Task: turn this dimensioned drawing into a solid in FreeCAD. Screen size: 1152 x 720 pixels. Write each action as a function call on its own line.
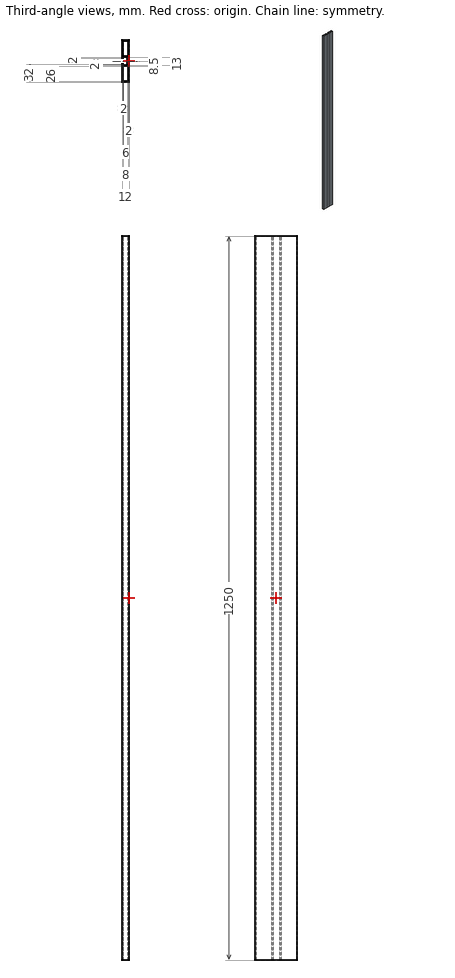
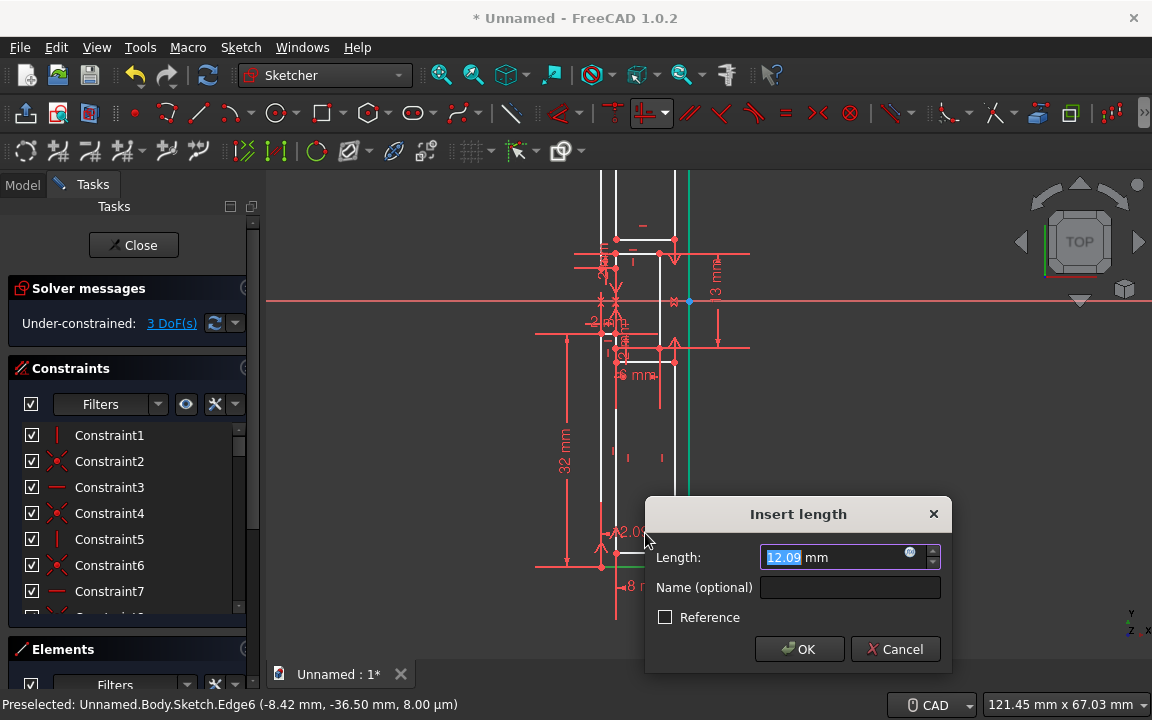
text(12)
key(Return)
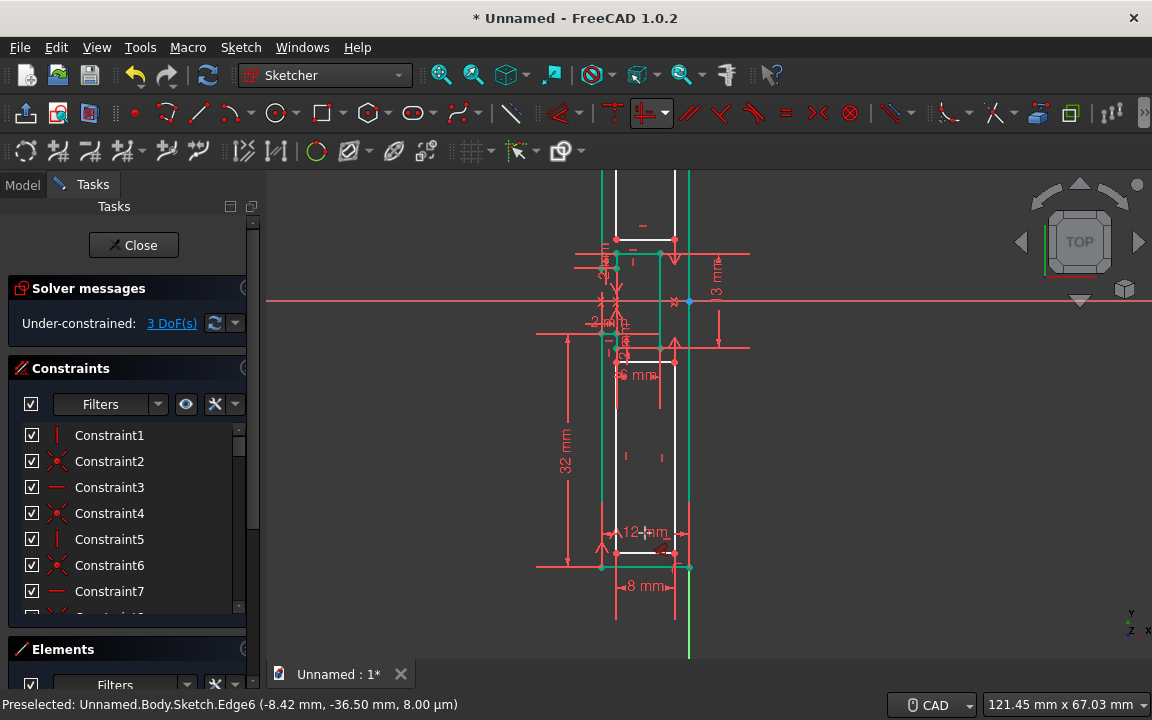
click(616, 420)
click(582, 414)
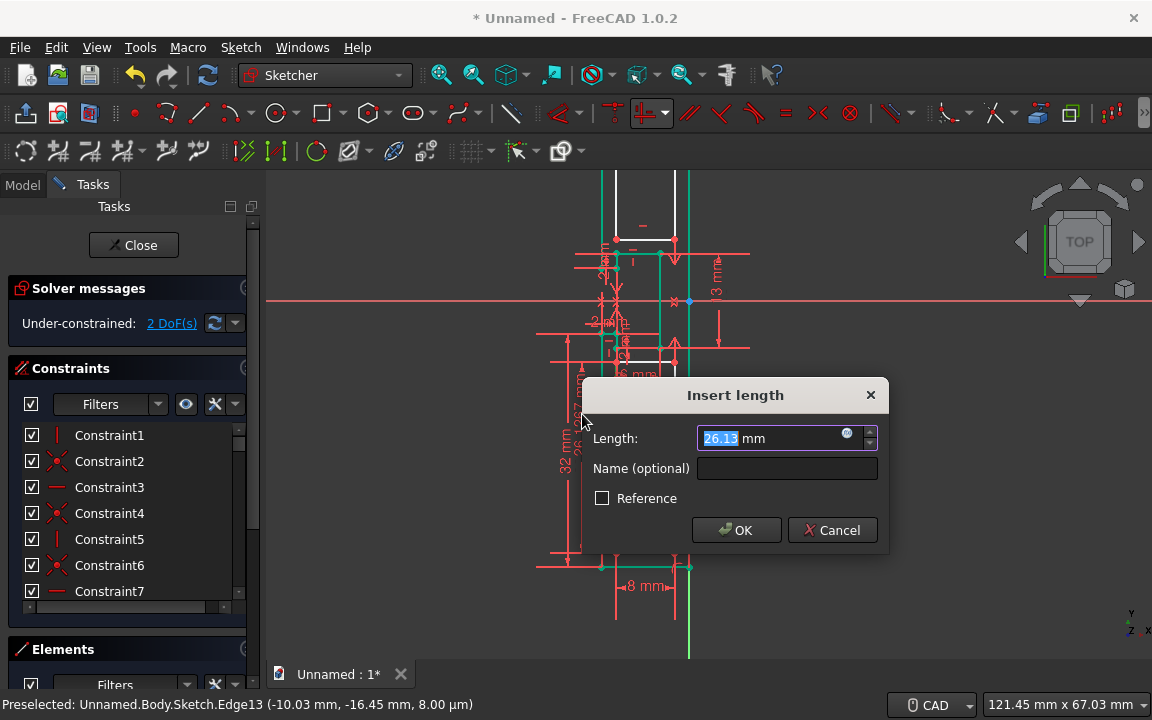
text(26)
key(Return)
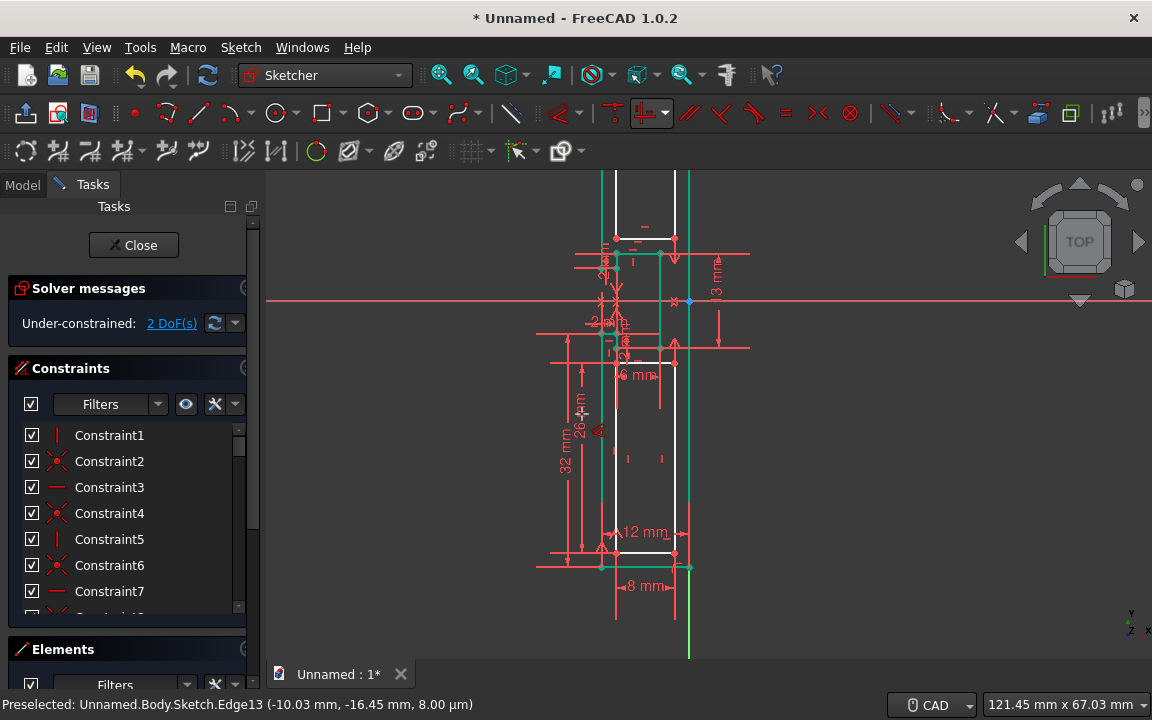
scroll(675, 553, up, 6)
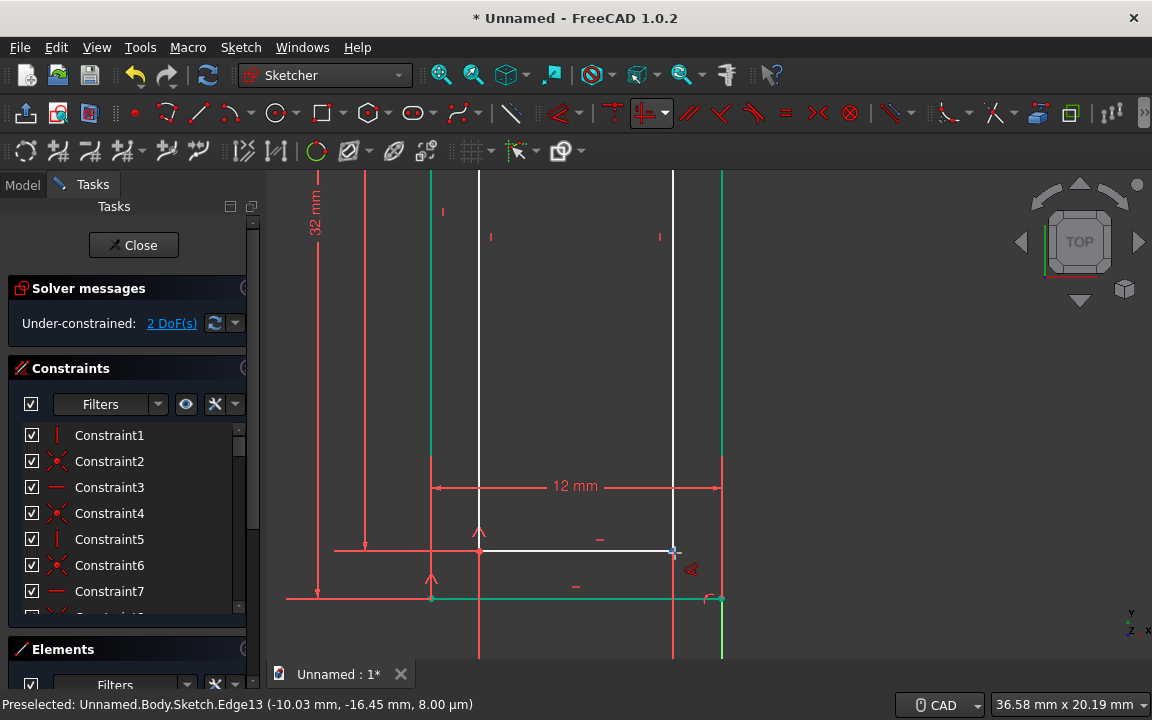
click(673, 551)
click(697, 585)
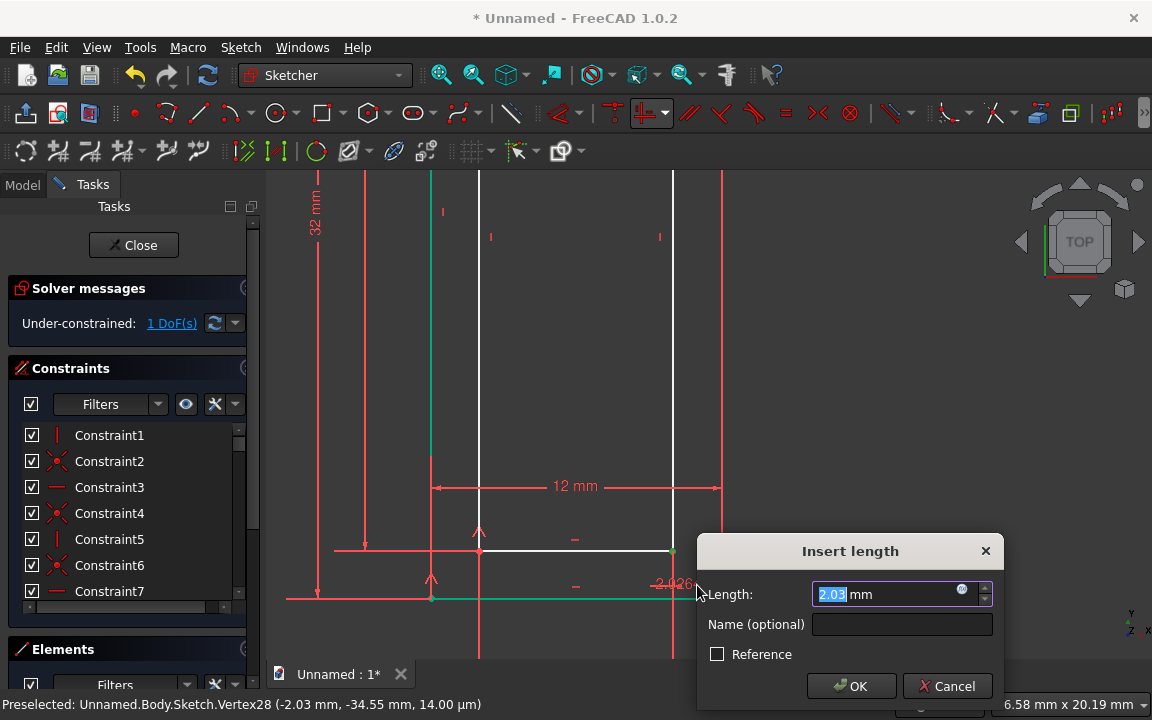
text(2)
key(Return)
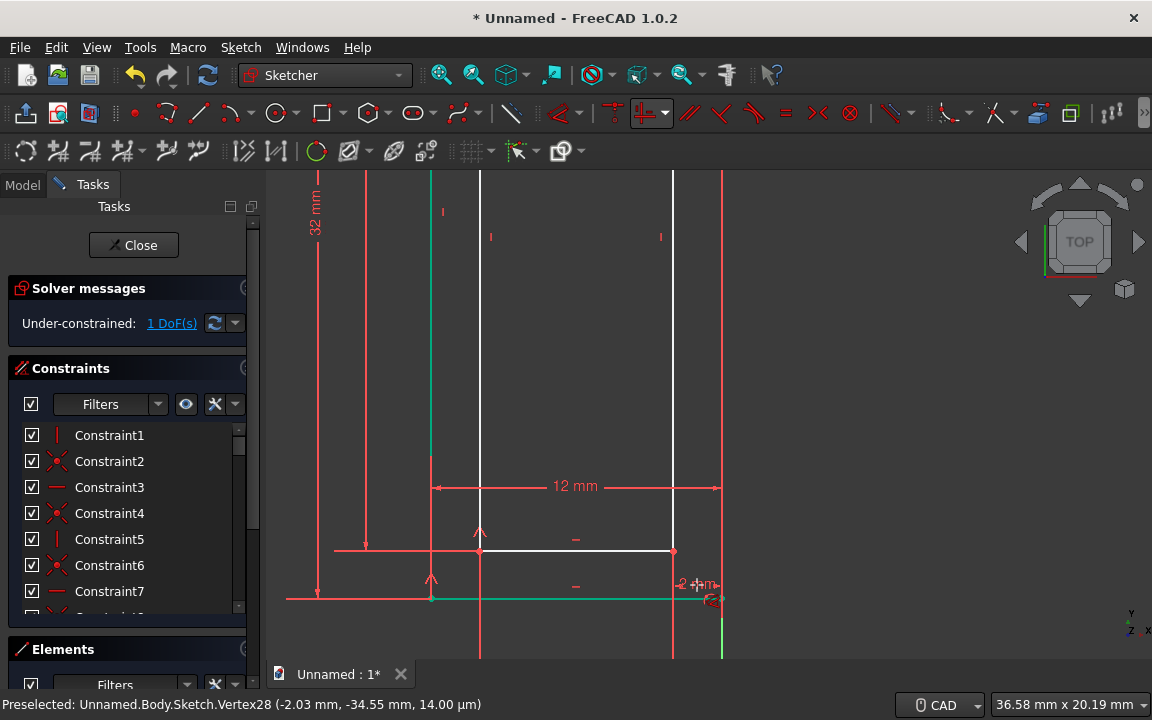
scroll(653, 553, down, 9)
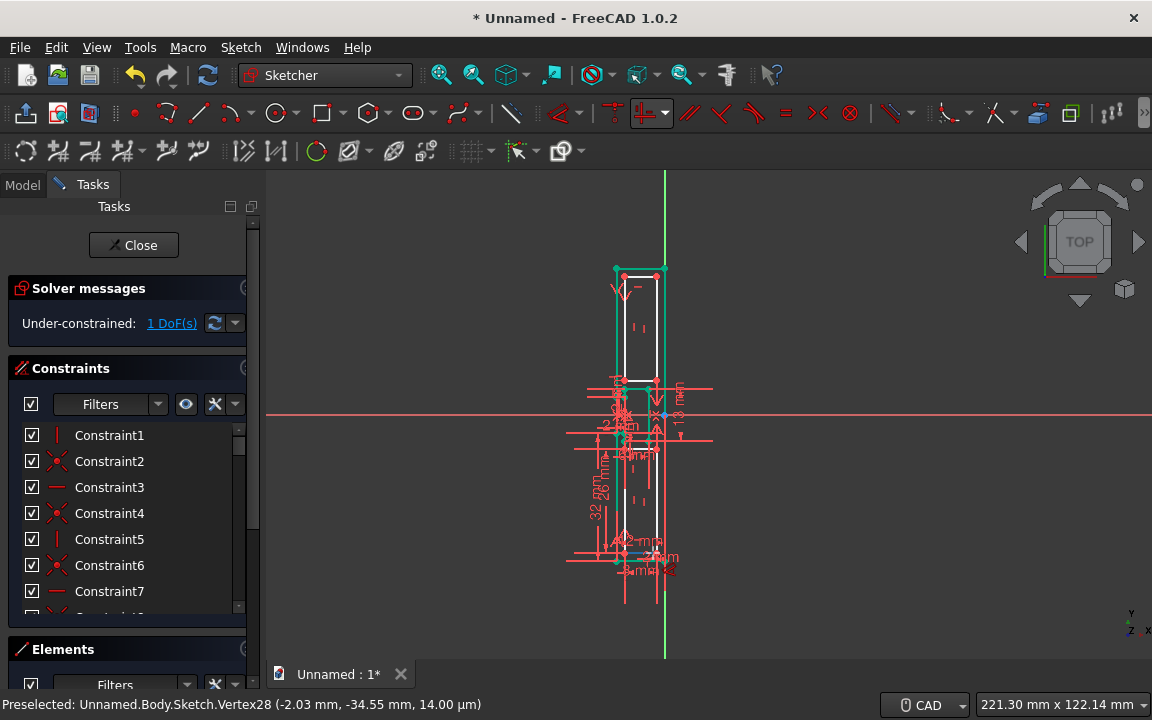
scroll(625, 449, up, 2)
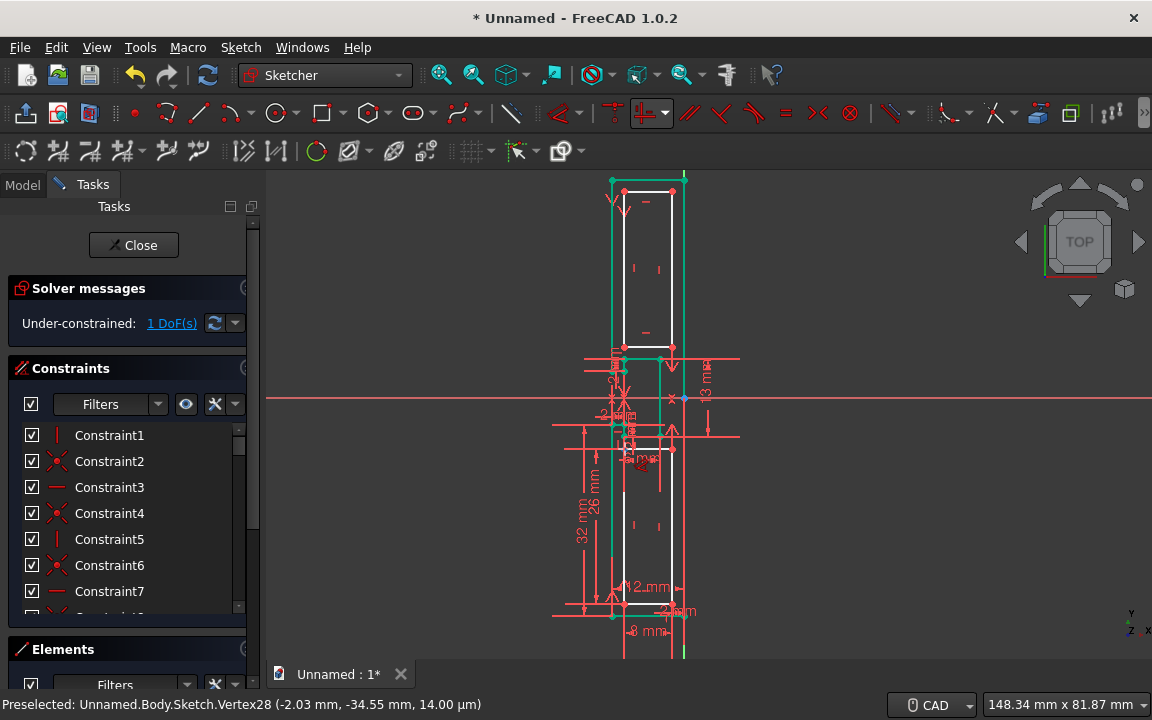
click(624, 449)
click(718, 424)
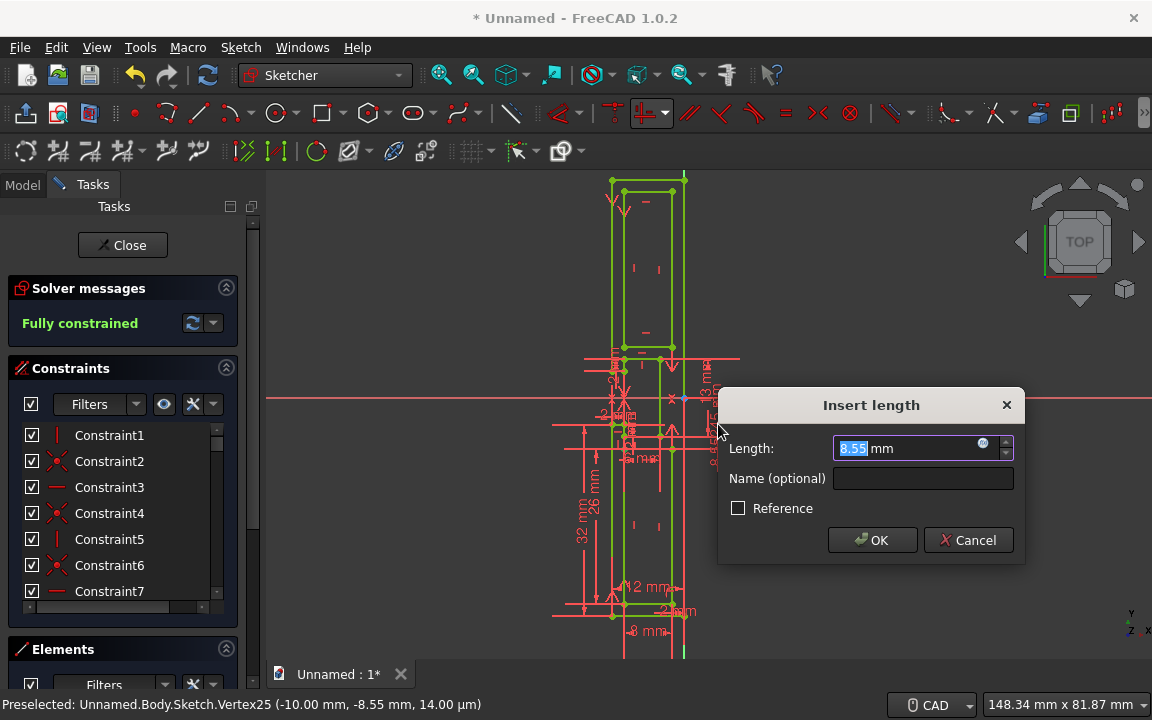
text(8.5)
key(Return)
key(Escape)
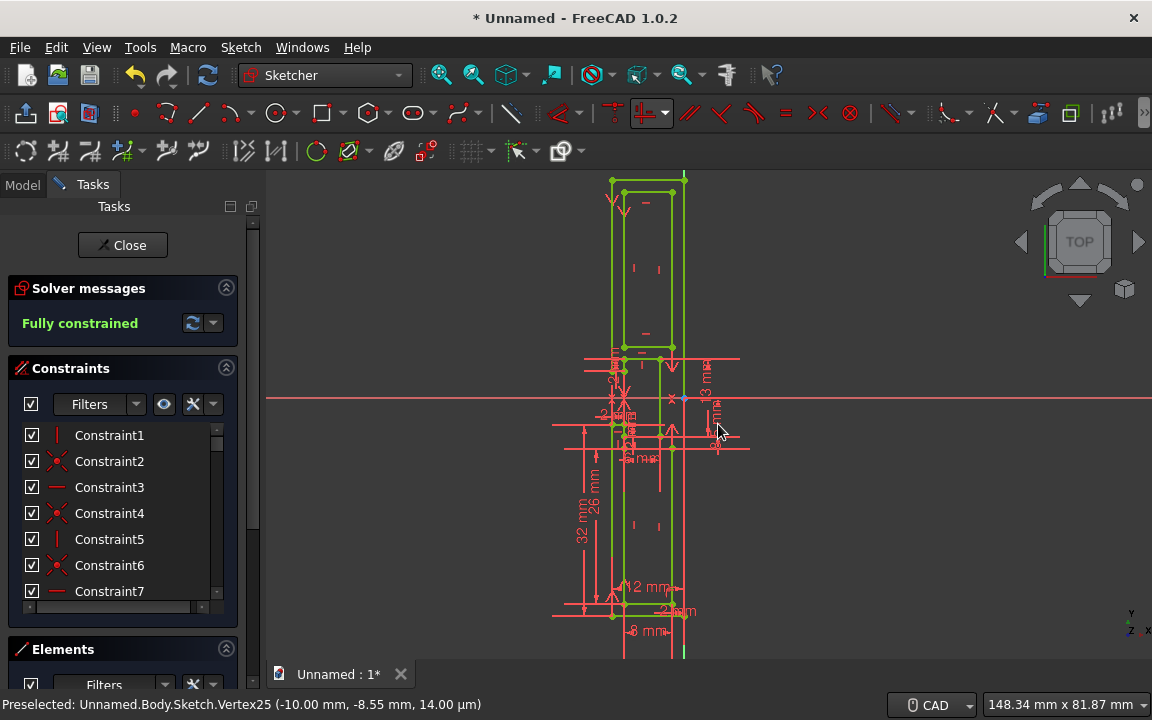
click(123, 245)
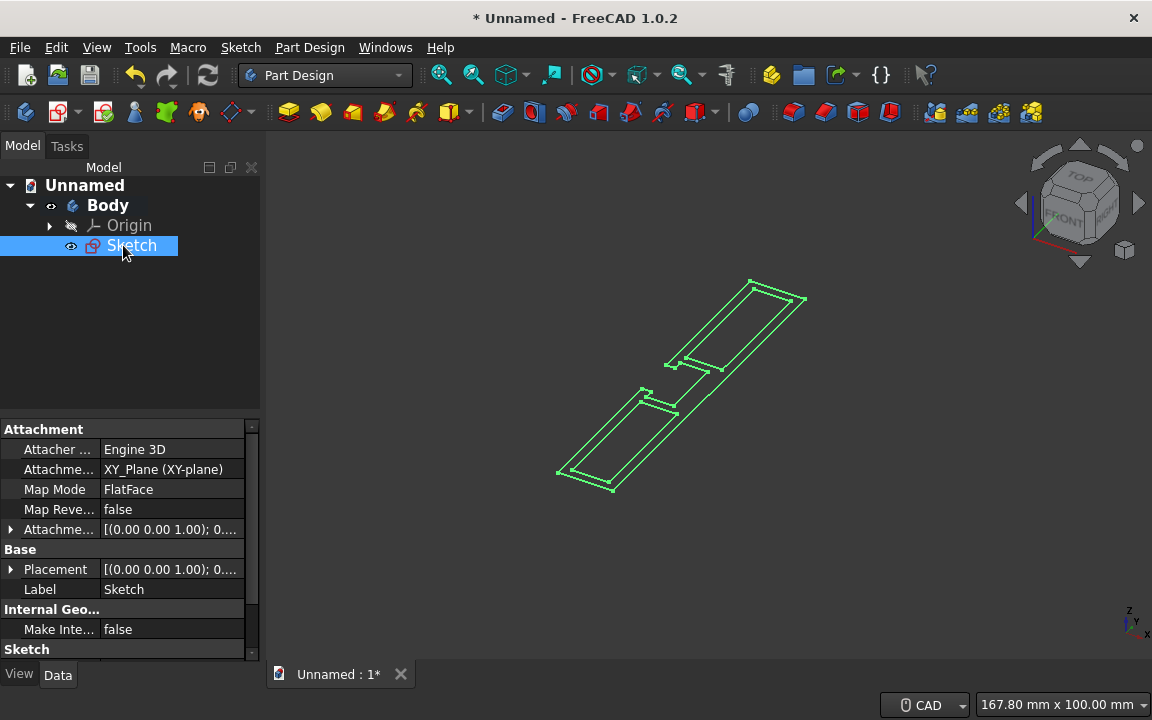
click(290, 112)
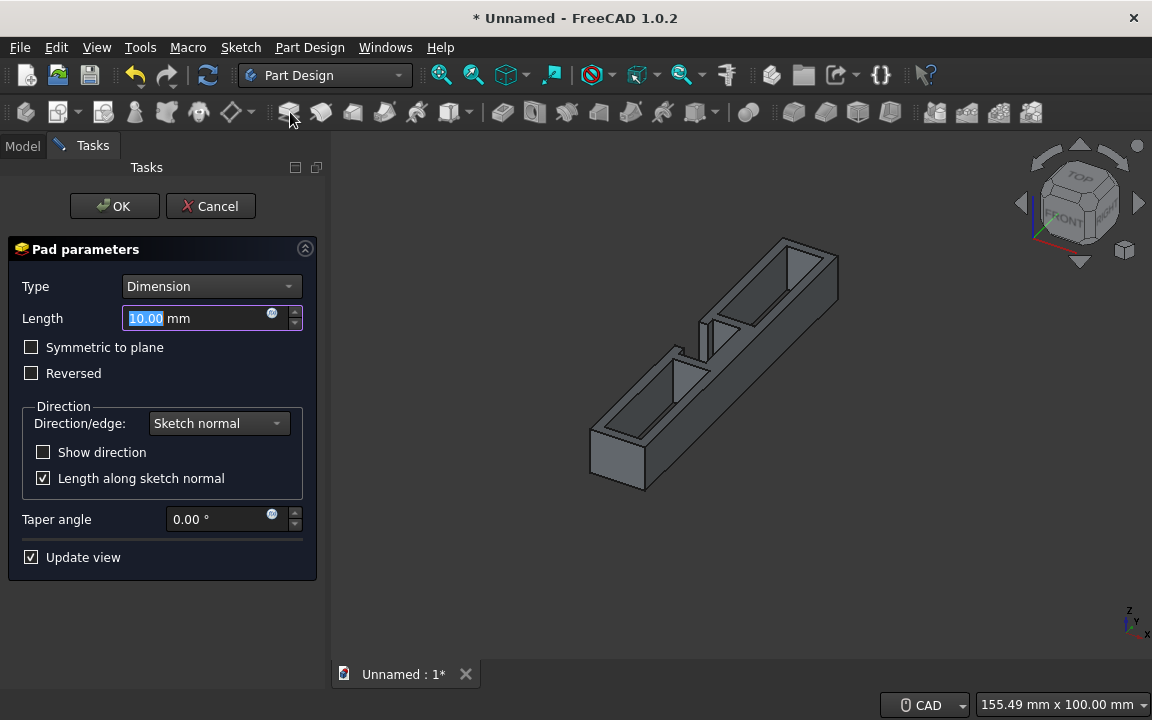
text(1250)
key(Tab)